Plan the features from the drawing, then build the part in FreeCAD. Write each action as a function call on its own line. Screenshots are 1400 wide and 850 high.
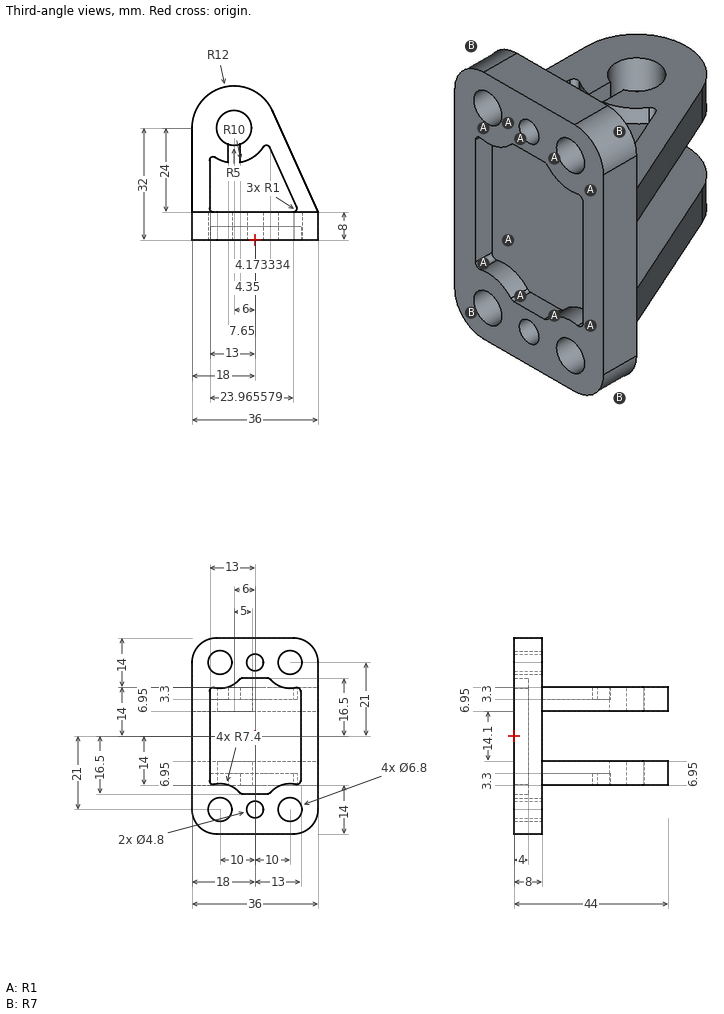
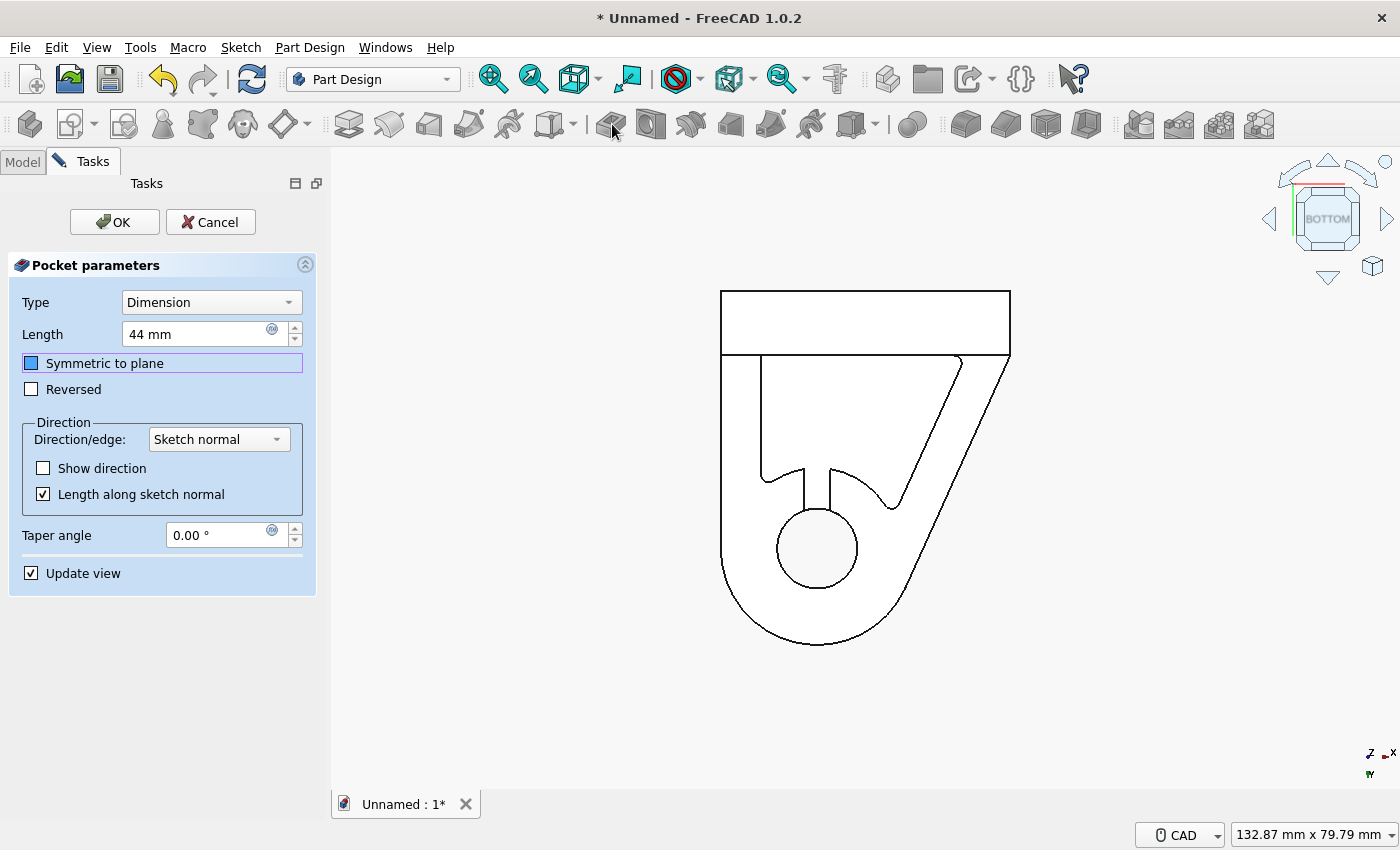
click(115, 222)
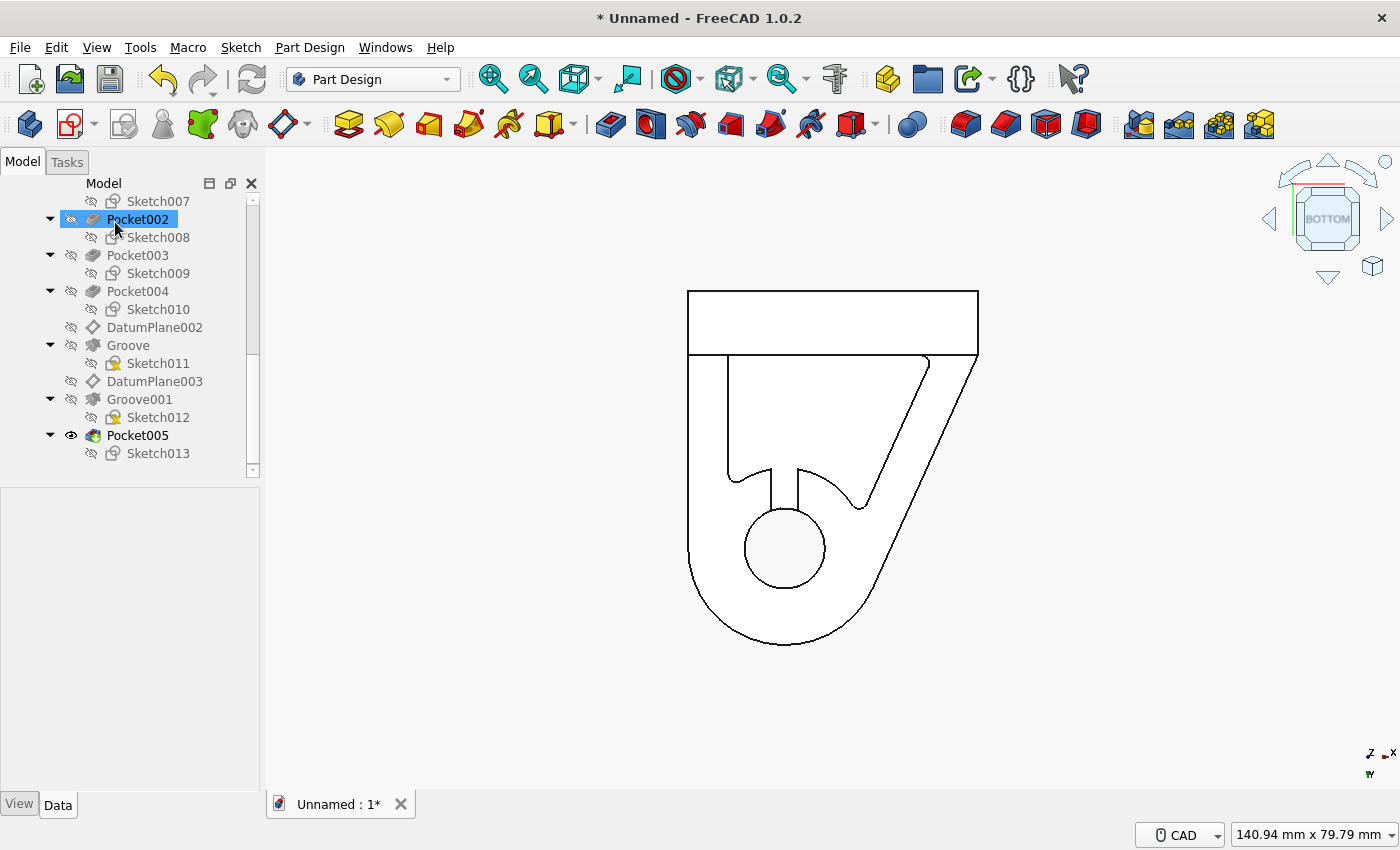
click(70, 124)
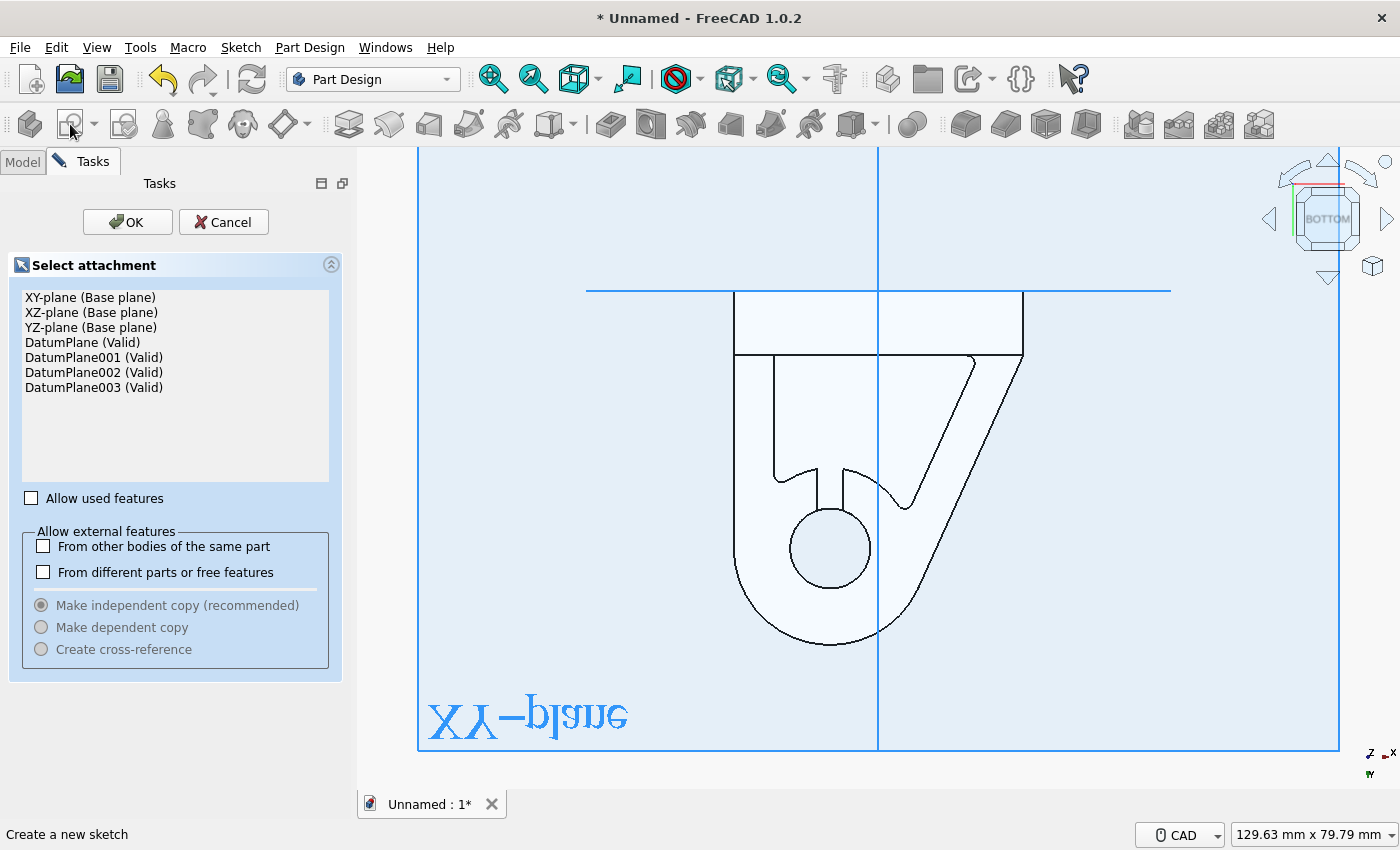
click(82, 312)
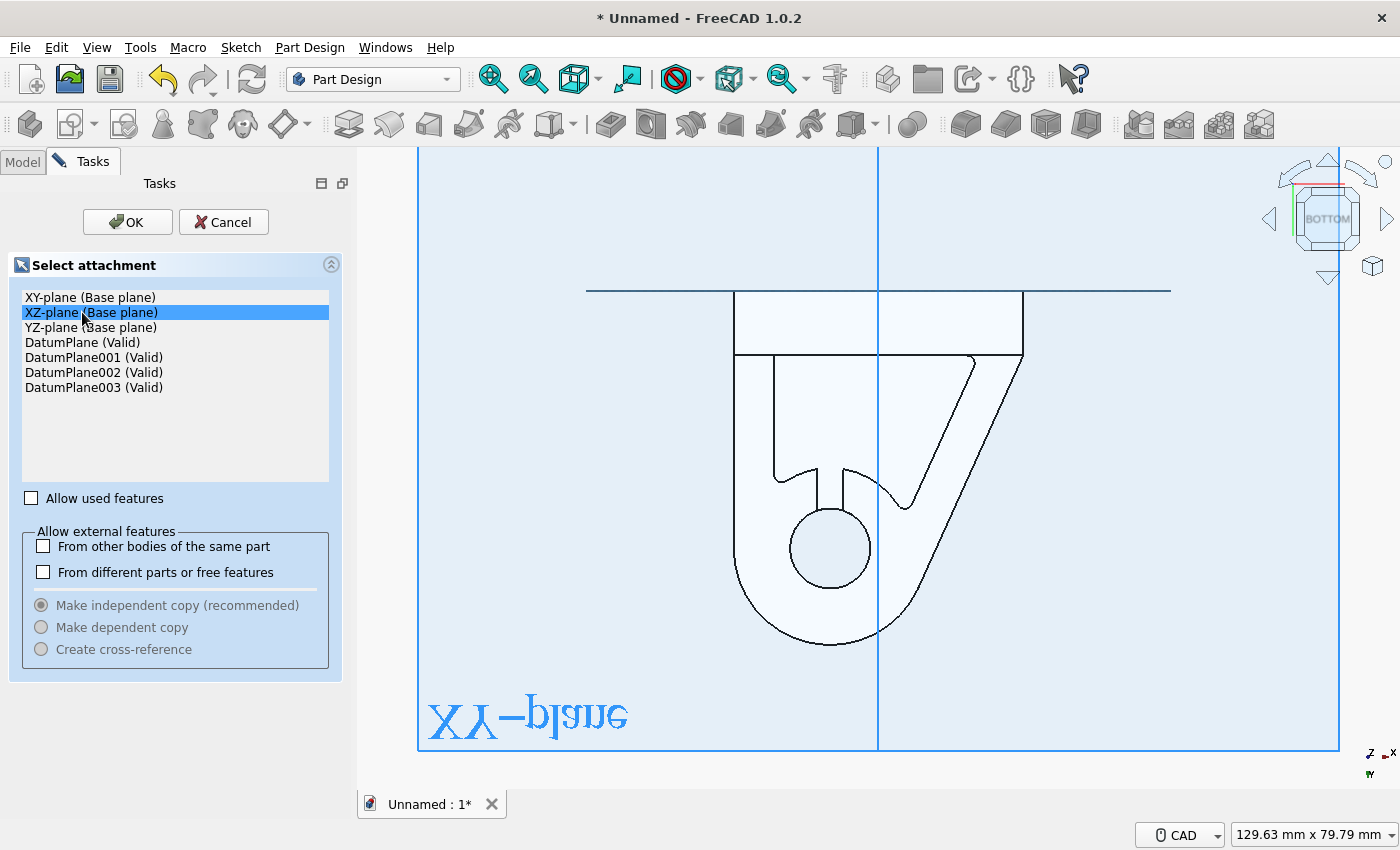
click(128, 222)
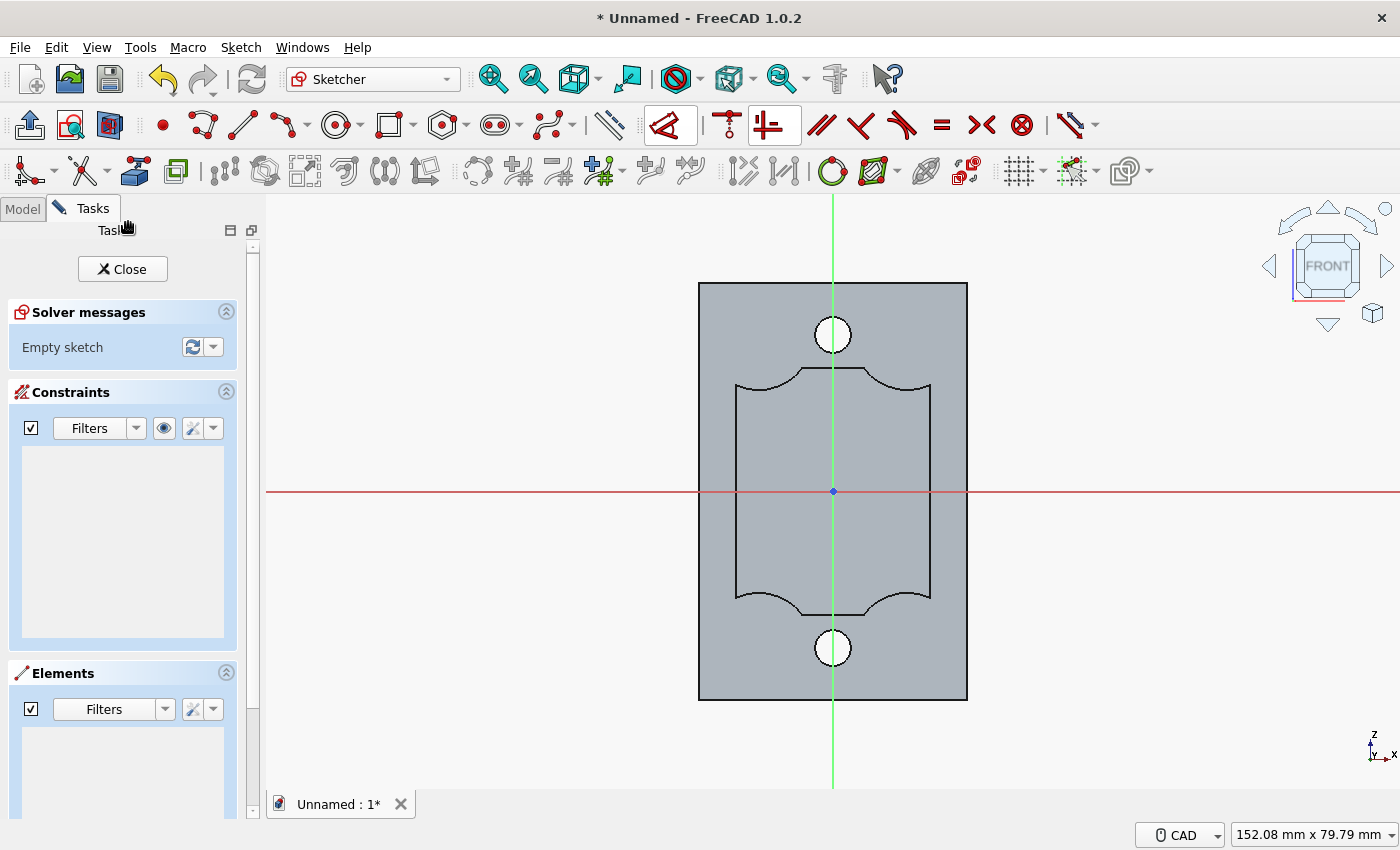
key(g)
key(c)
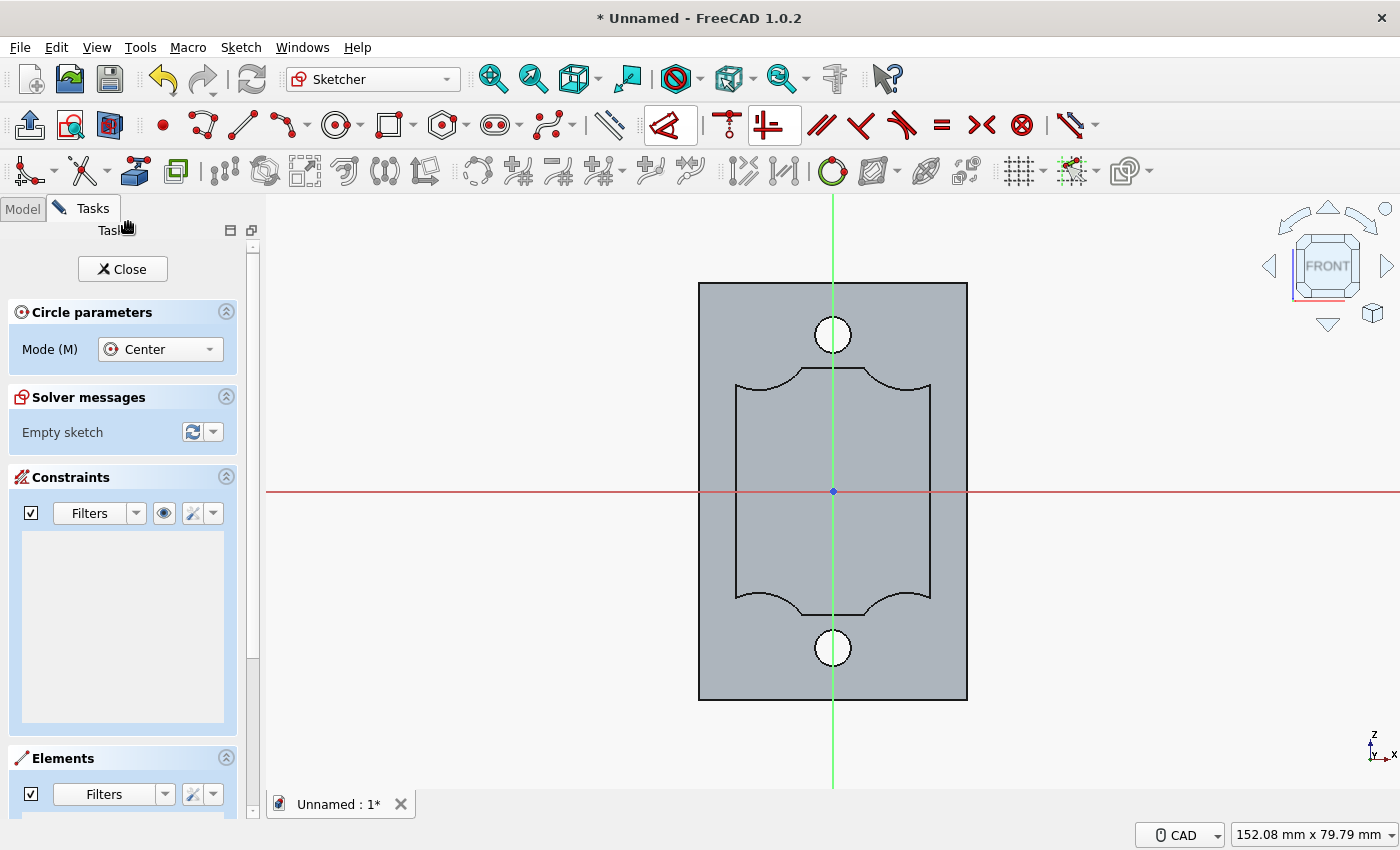
click(908, 648)
move(925, 630)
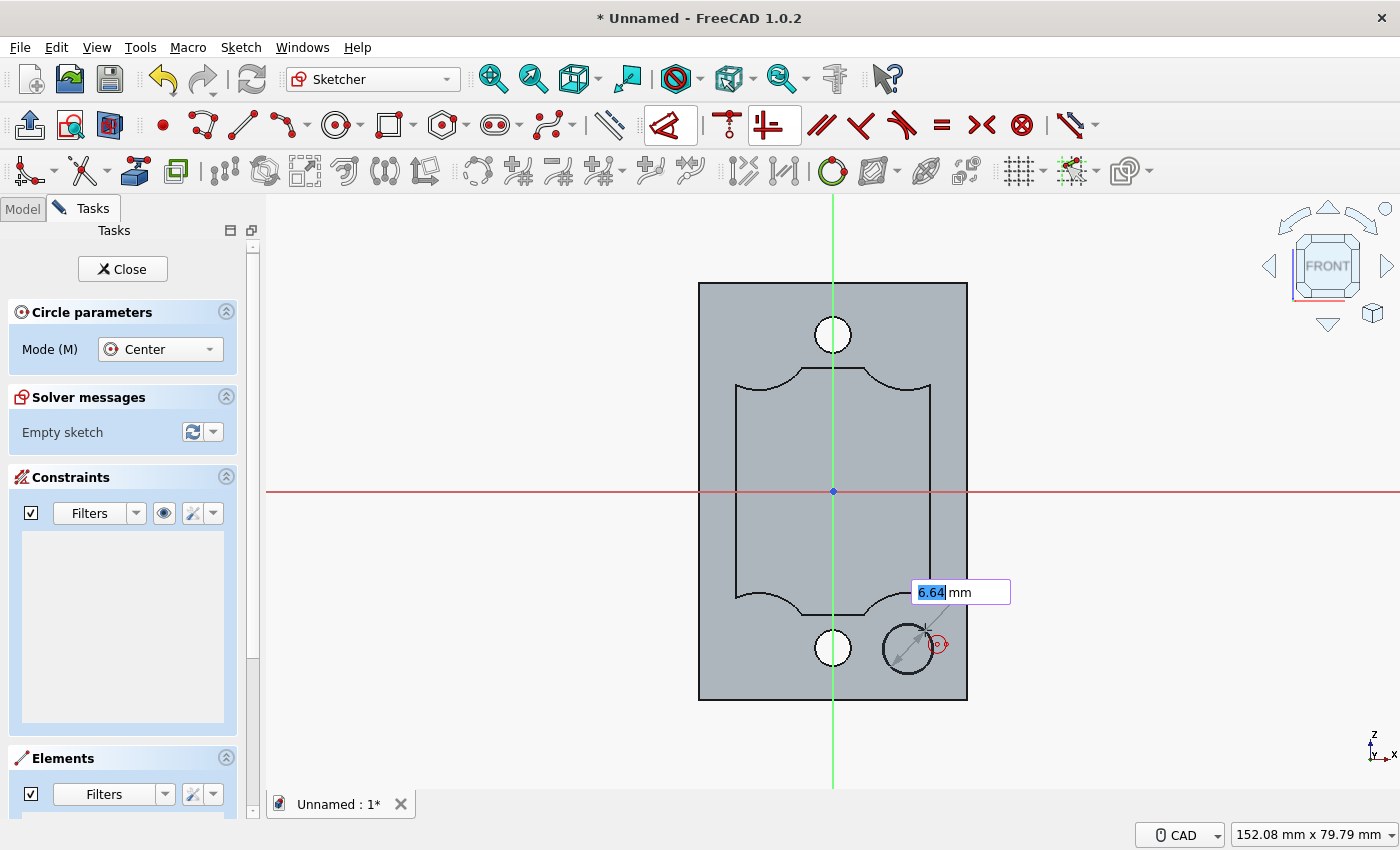
text(6.8)
key(Return)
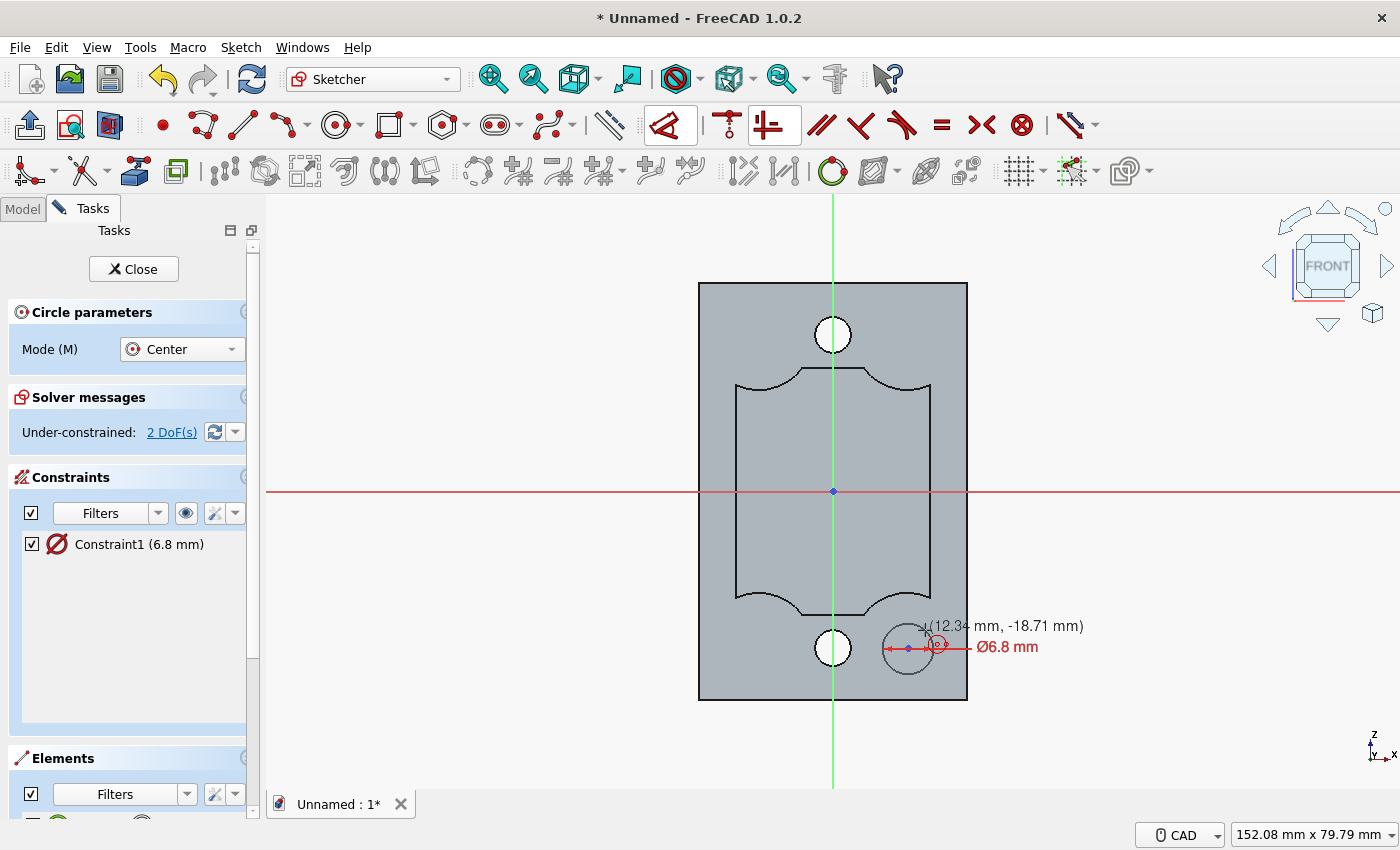
click(908, 335)
move(925, 317)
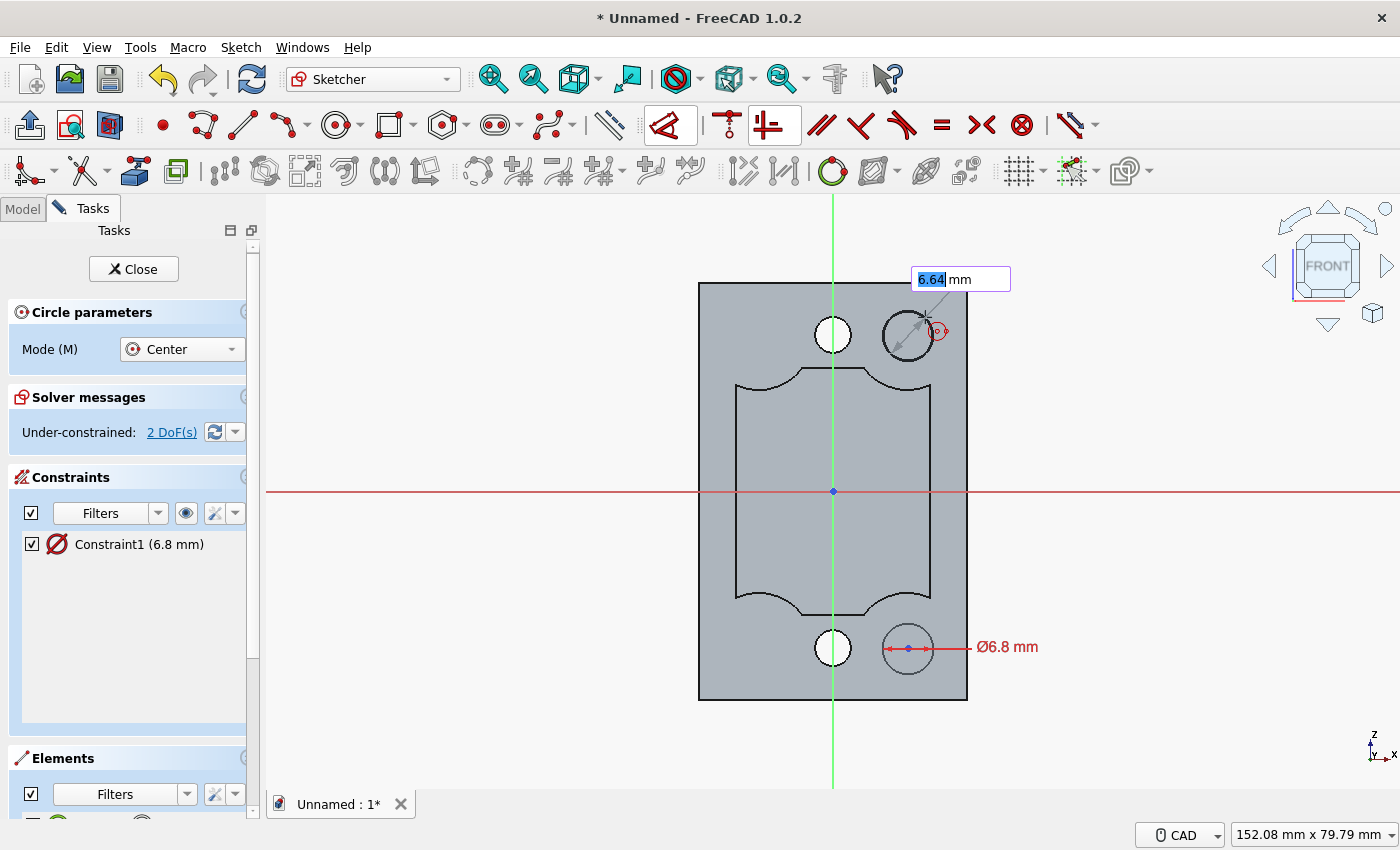
text(6.8)
key(Return)